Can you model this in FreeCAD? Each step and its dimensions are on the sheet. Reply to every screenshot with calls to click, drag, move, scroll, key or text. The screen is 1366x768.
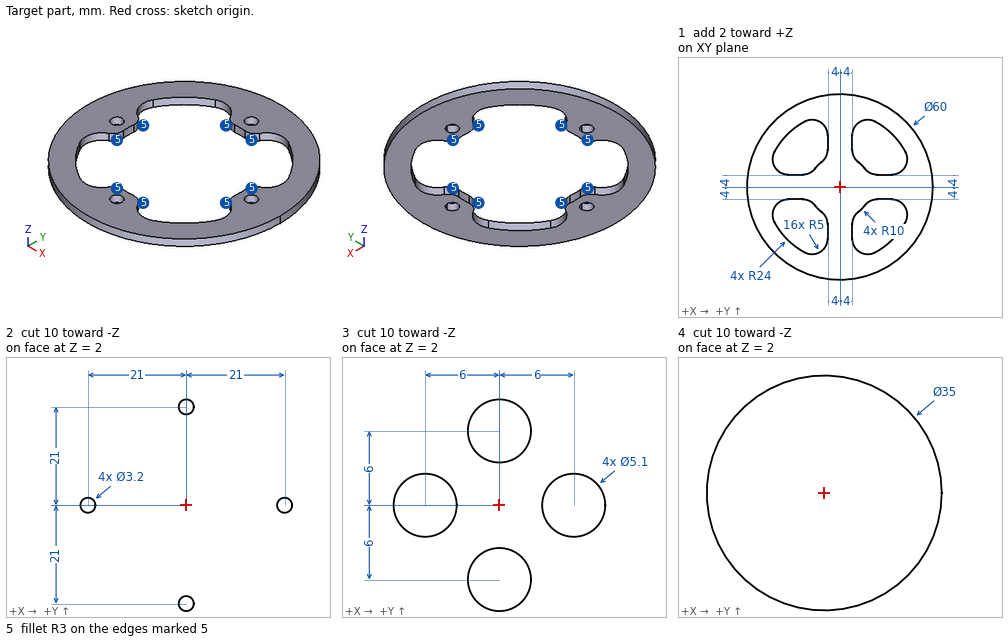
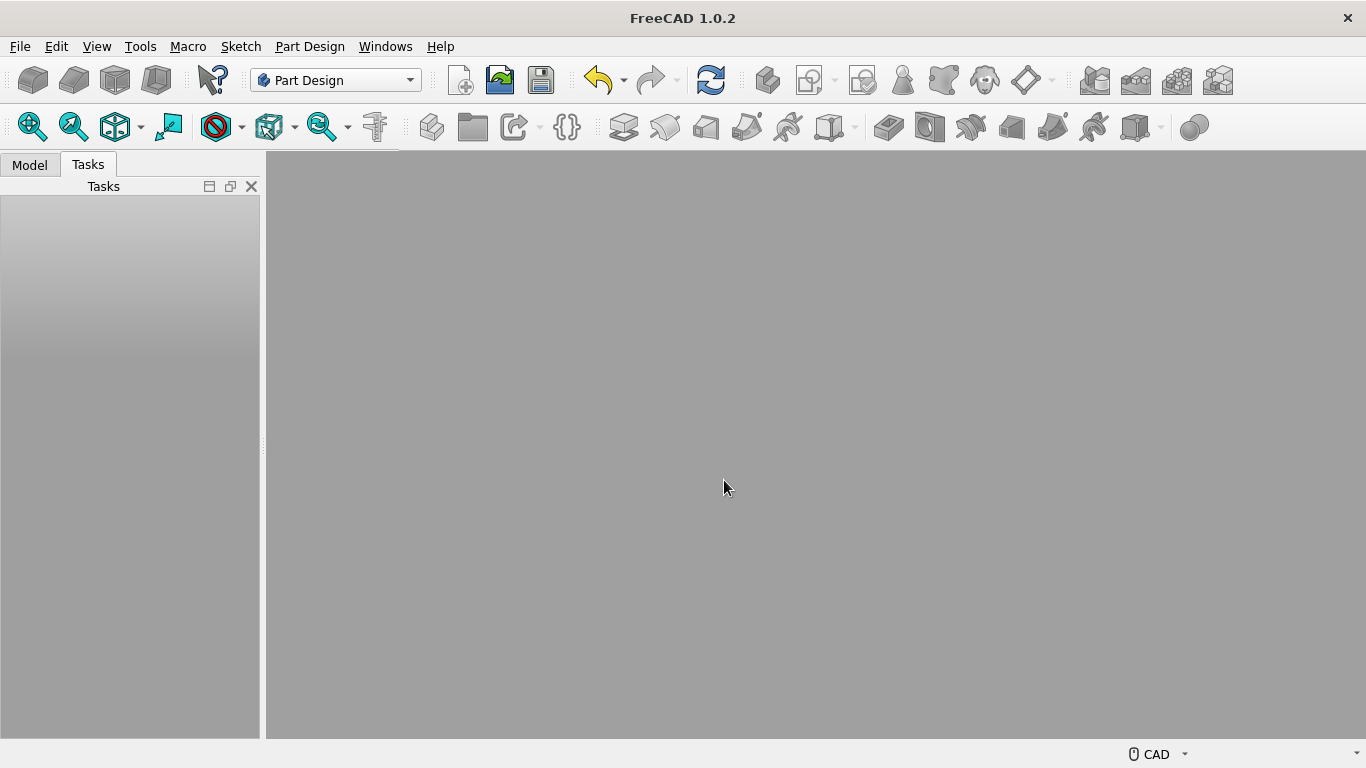
key(ctrl+n)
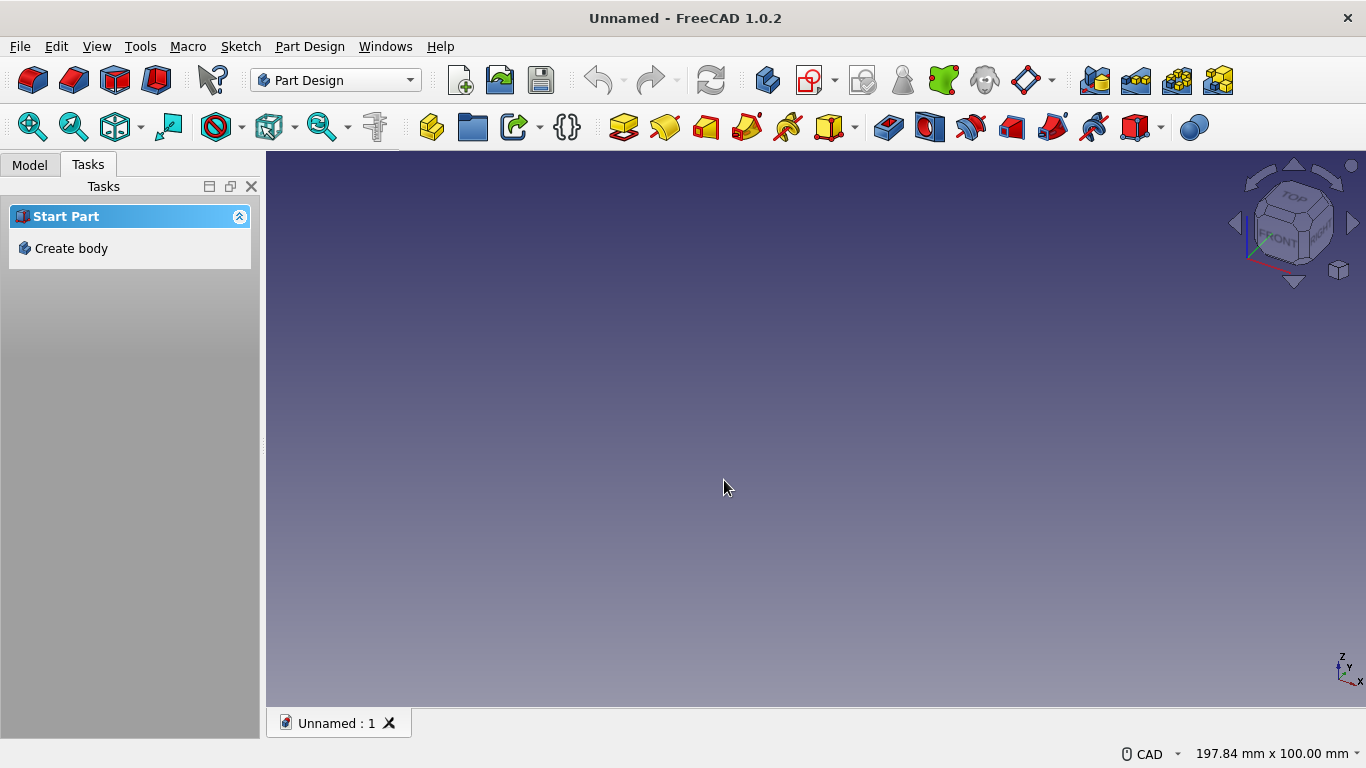
click(808, 80)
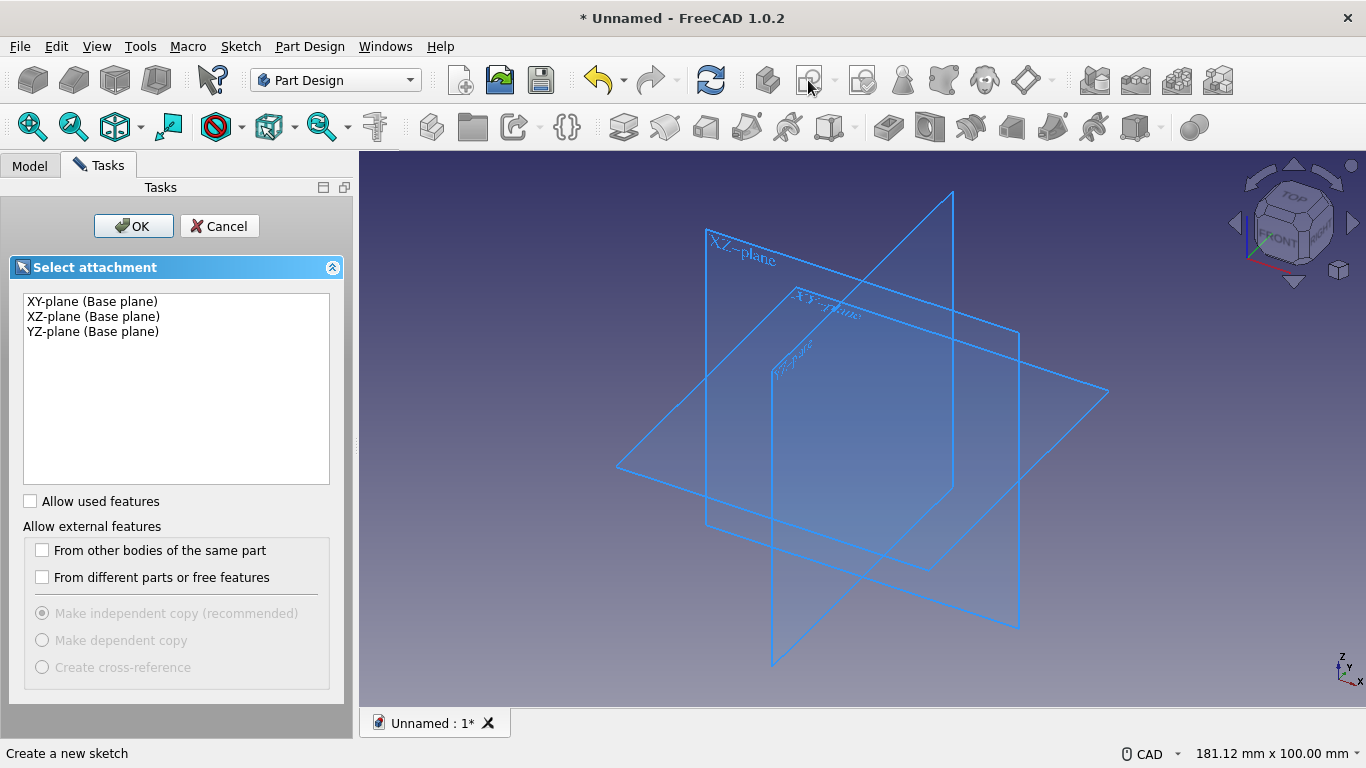
click(84, 302)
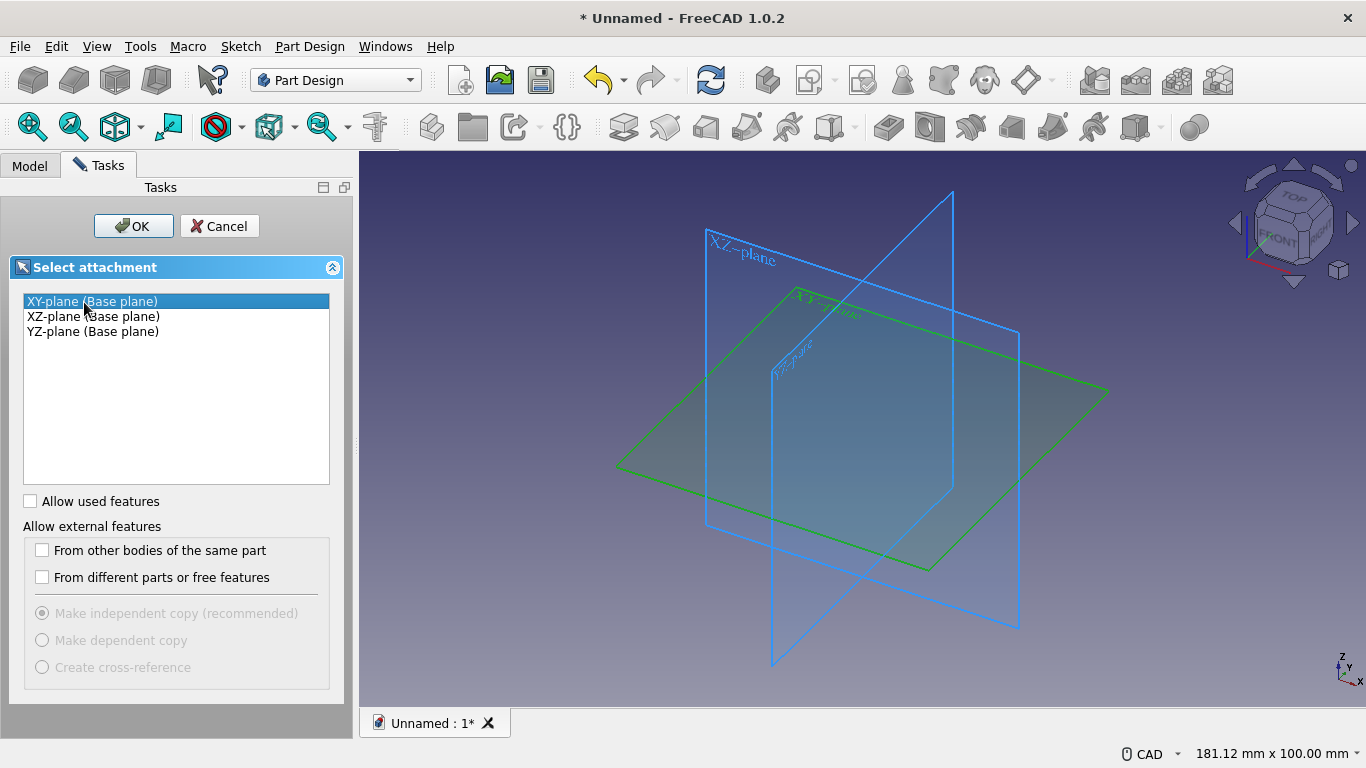
click(134, 226)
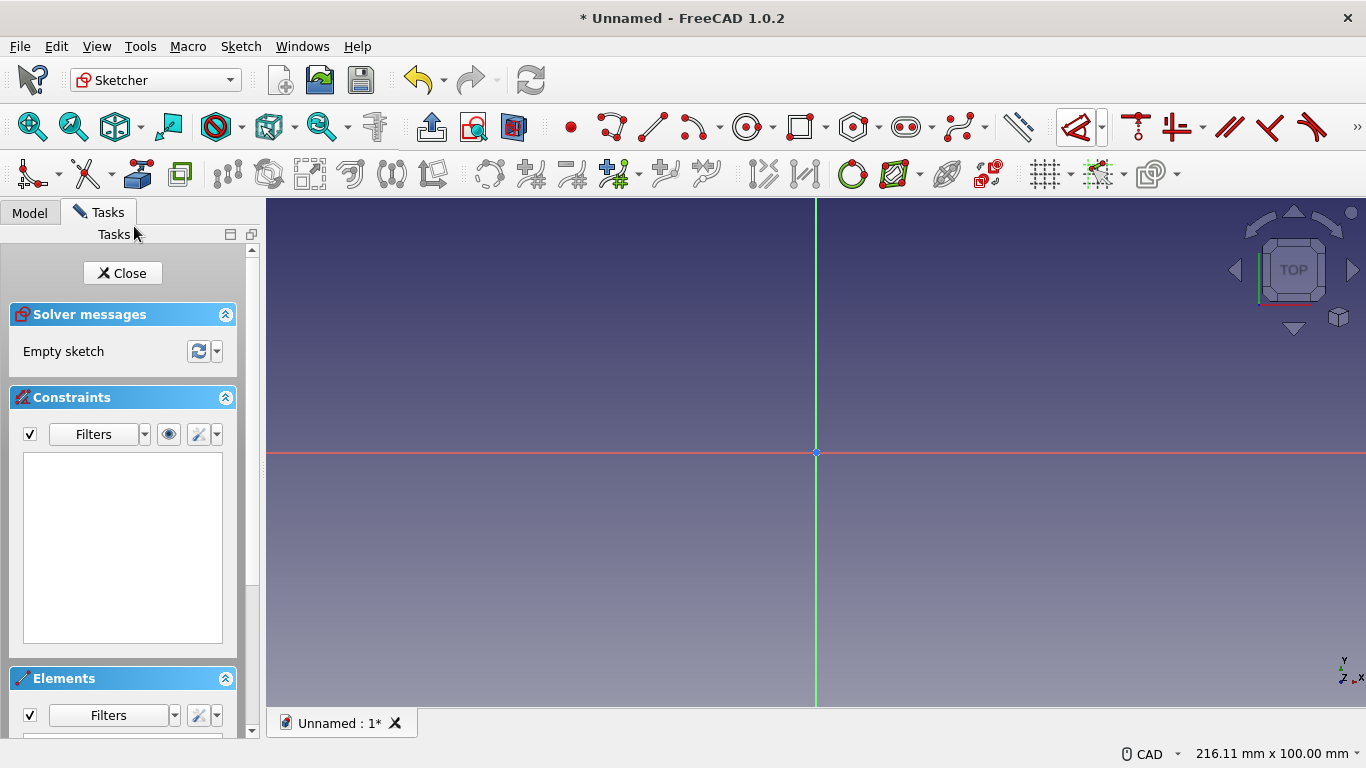
key(g)
key(l)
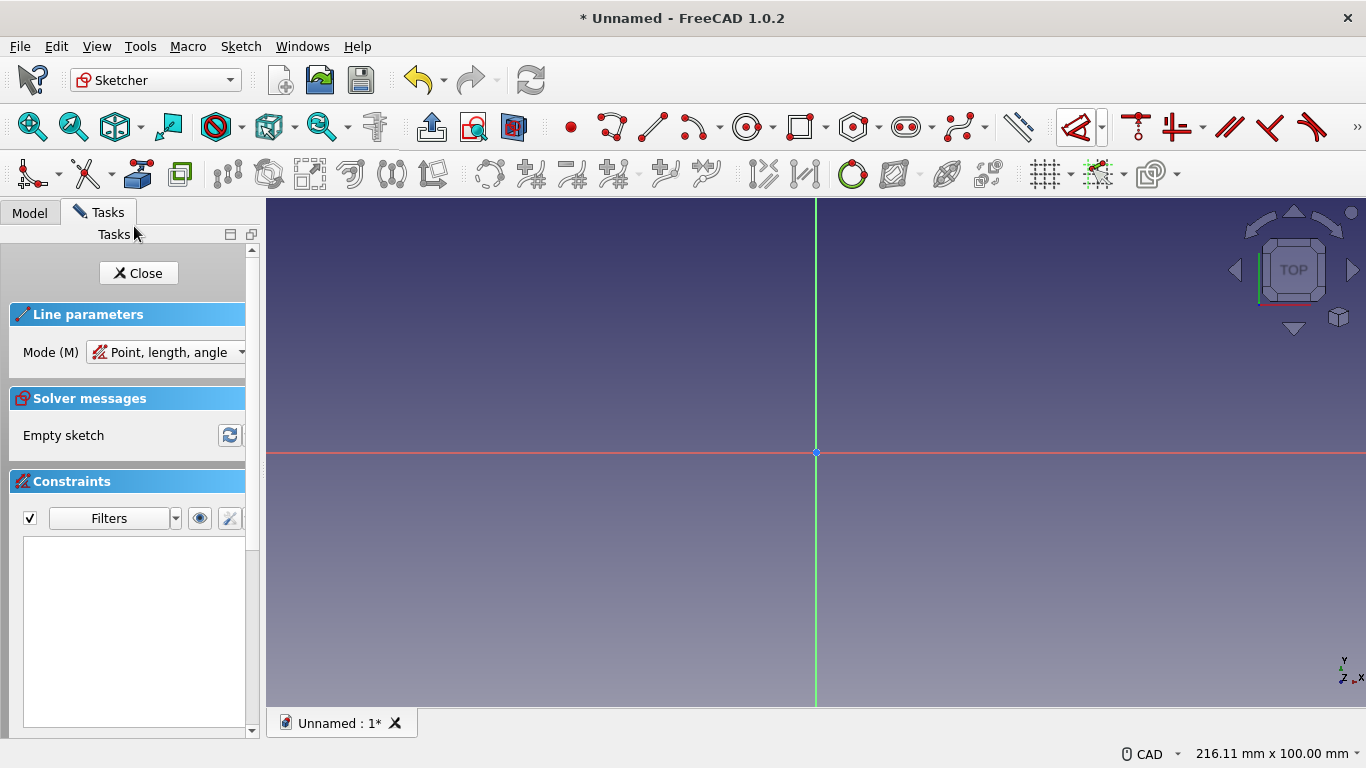
click(796, 514)
click(796, 538)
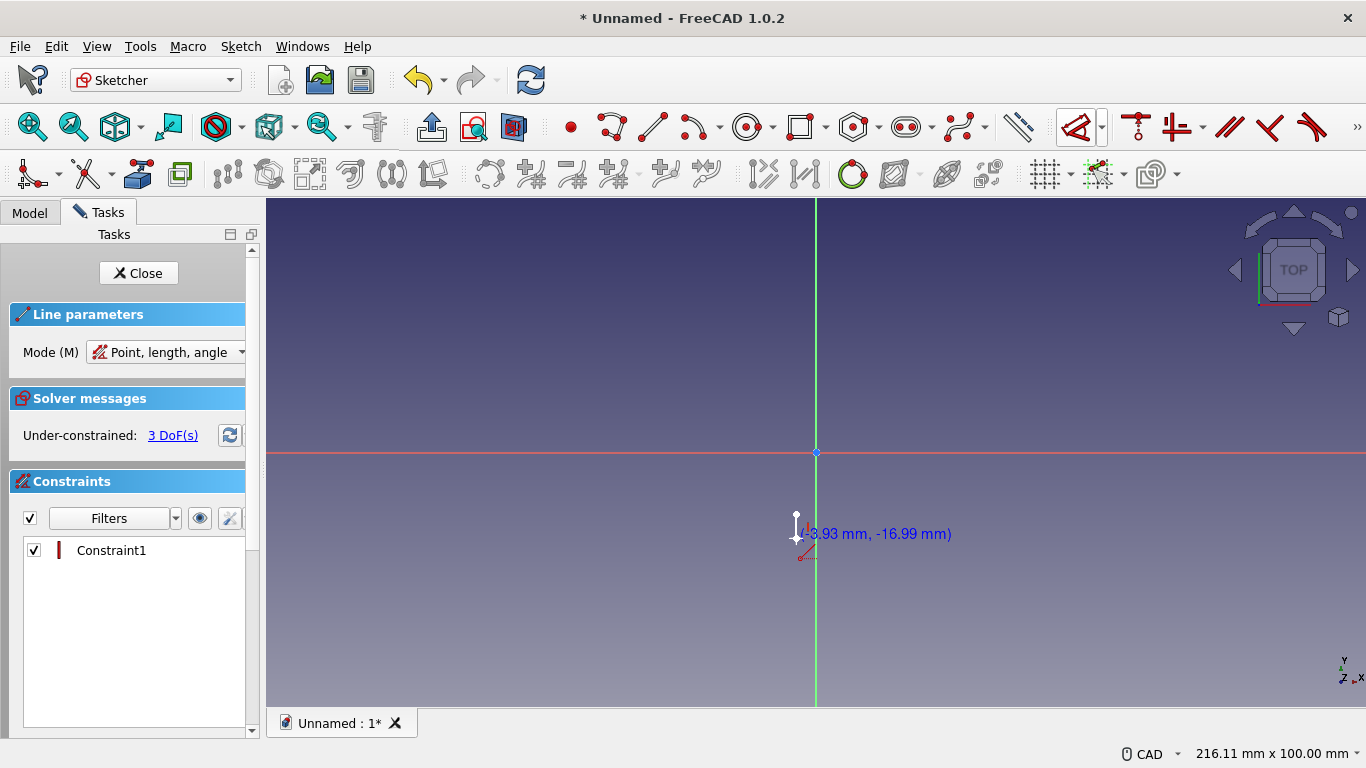
click(731, 473)
click(755, 473)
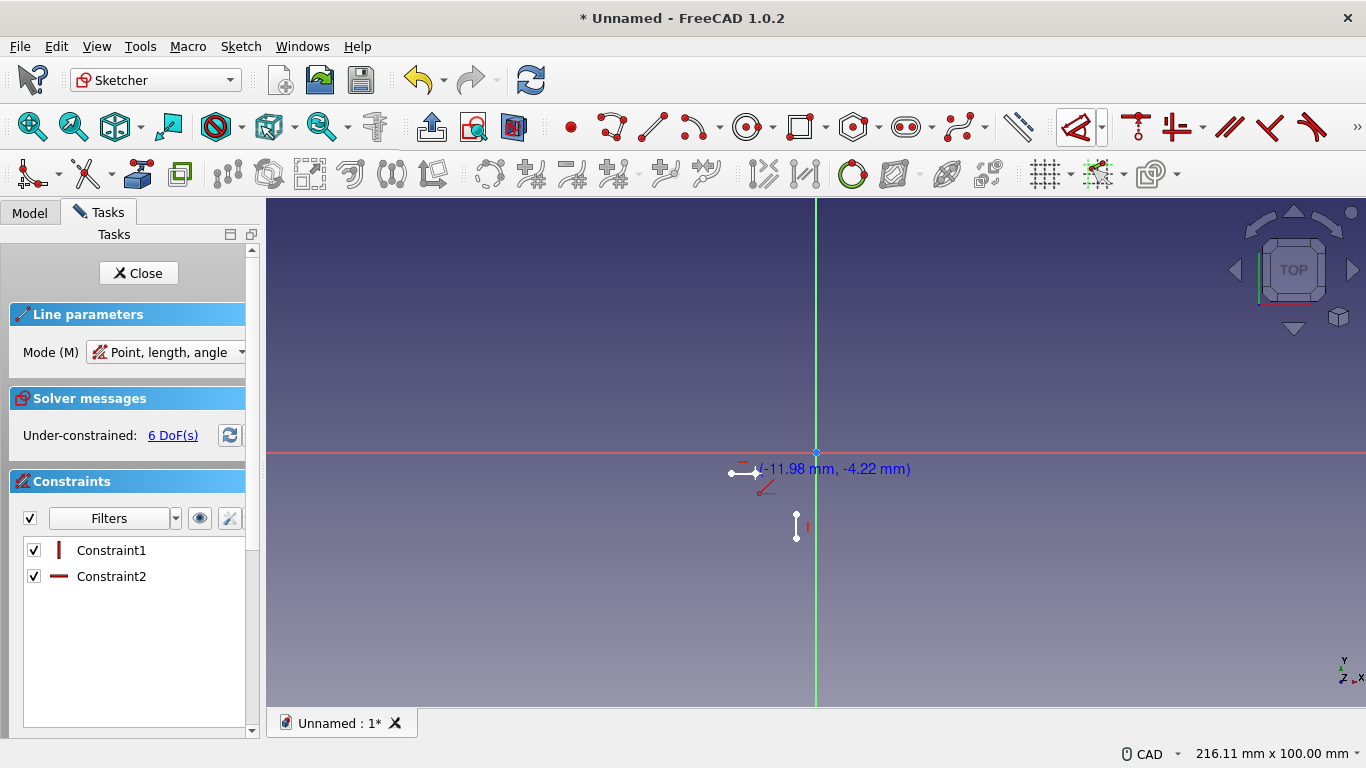
key(g)
key(3)
key(a)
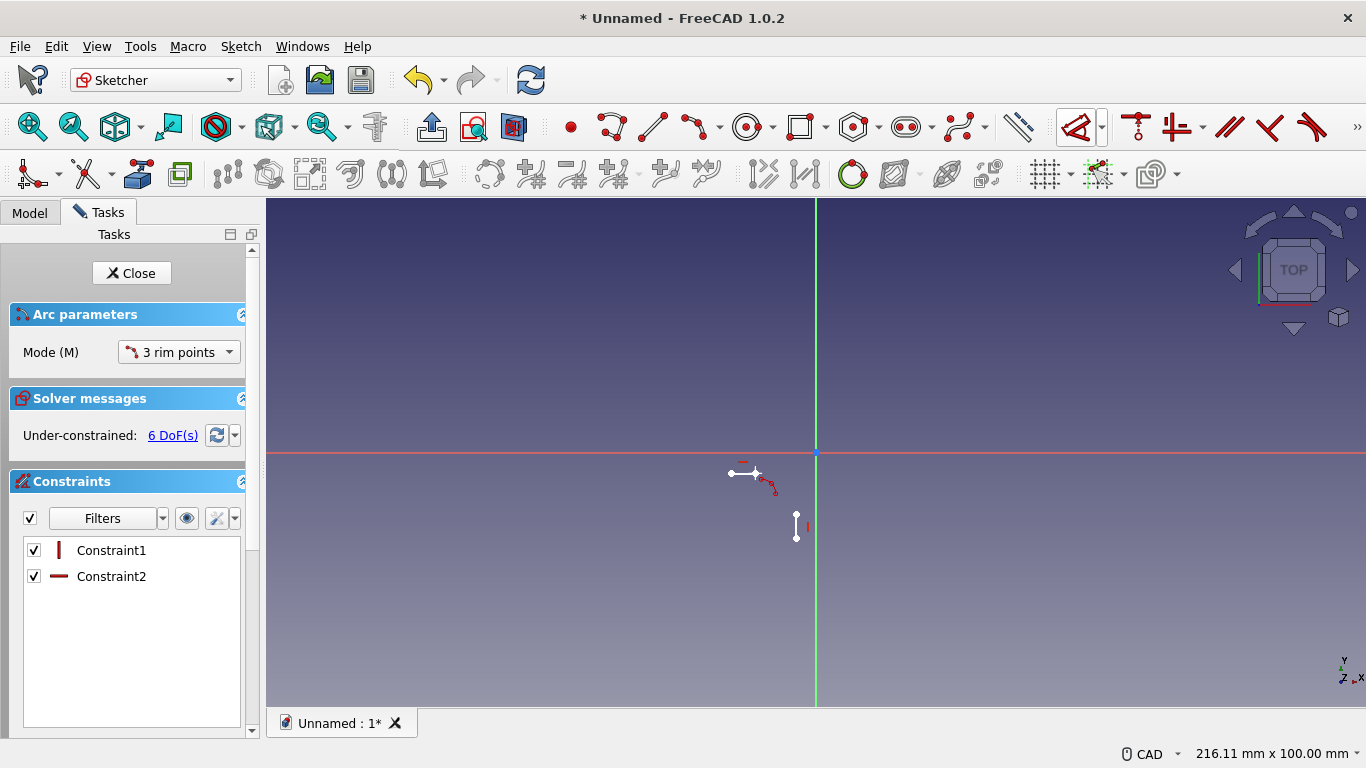
scroll(796, 538, up, 2)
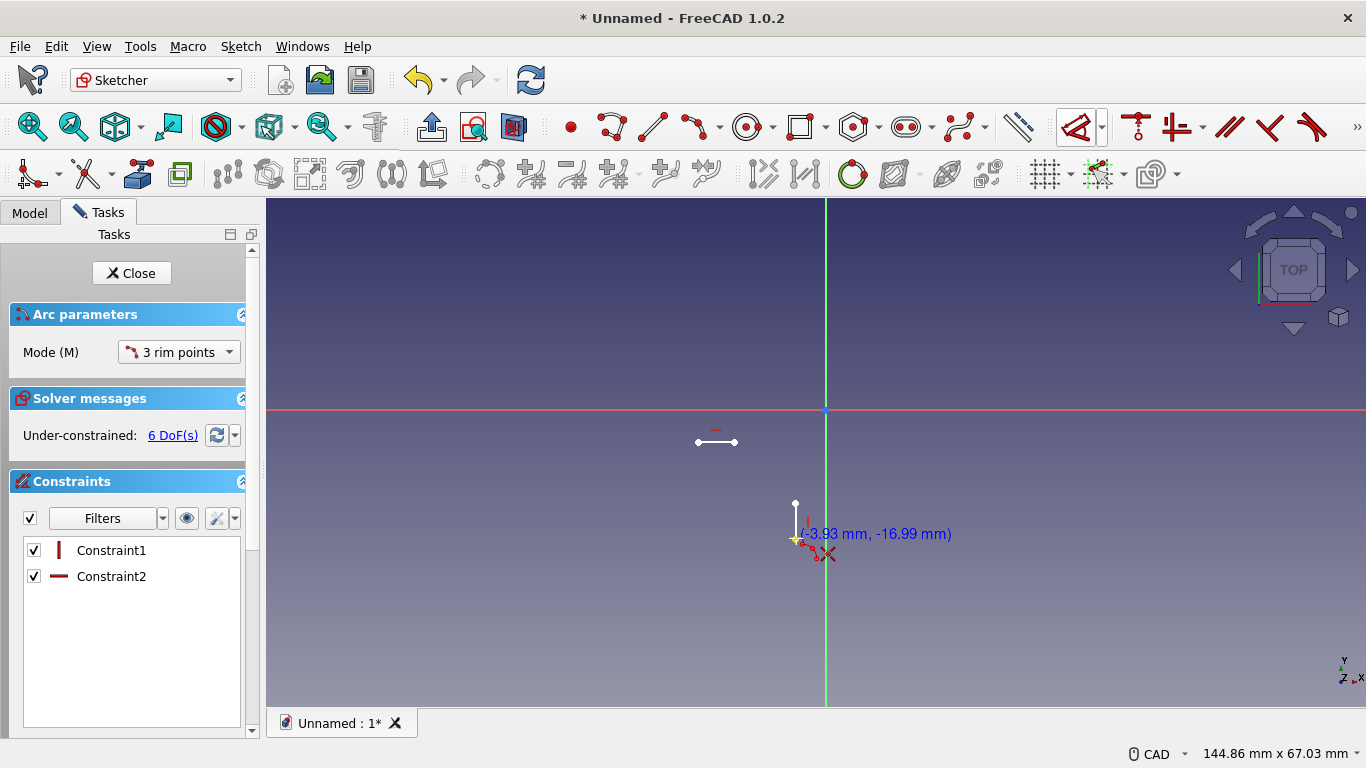
click(796, 539)
click(739, 571)
click(777, 570)